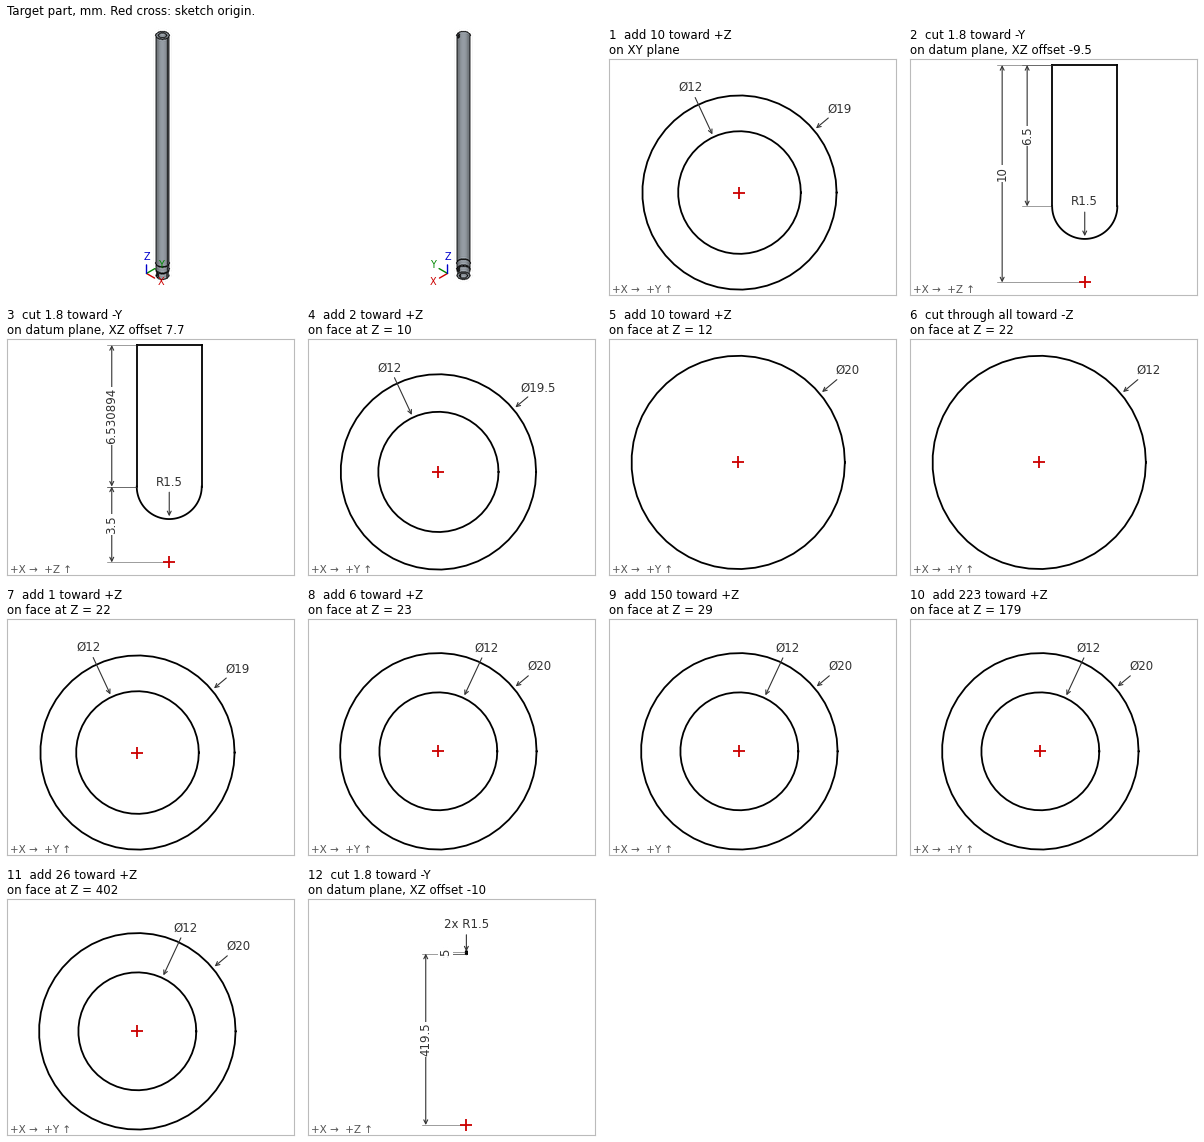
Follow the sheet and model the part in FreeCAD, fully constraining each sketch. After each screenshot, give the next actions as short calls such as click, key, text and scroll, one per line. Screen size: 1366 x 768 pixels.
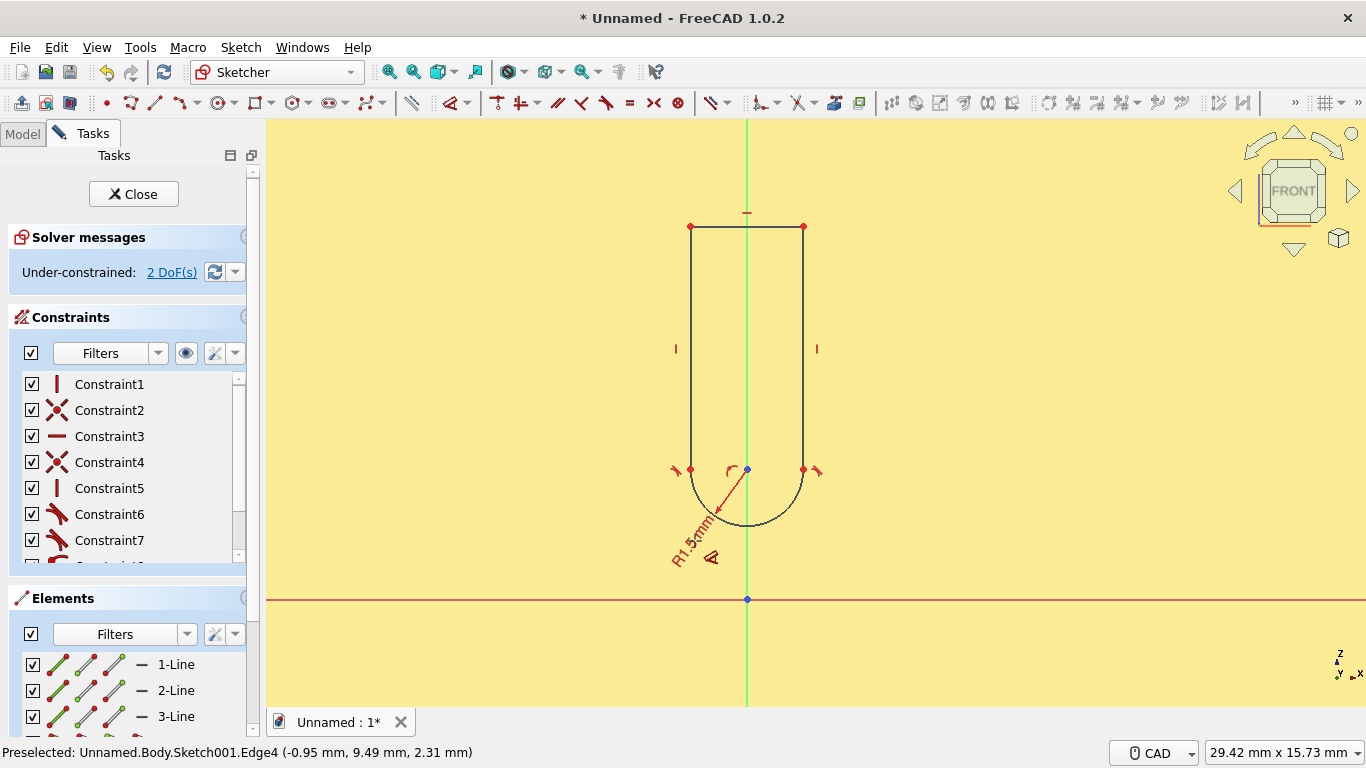
click(691, 397)
click(657, 349)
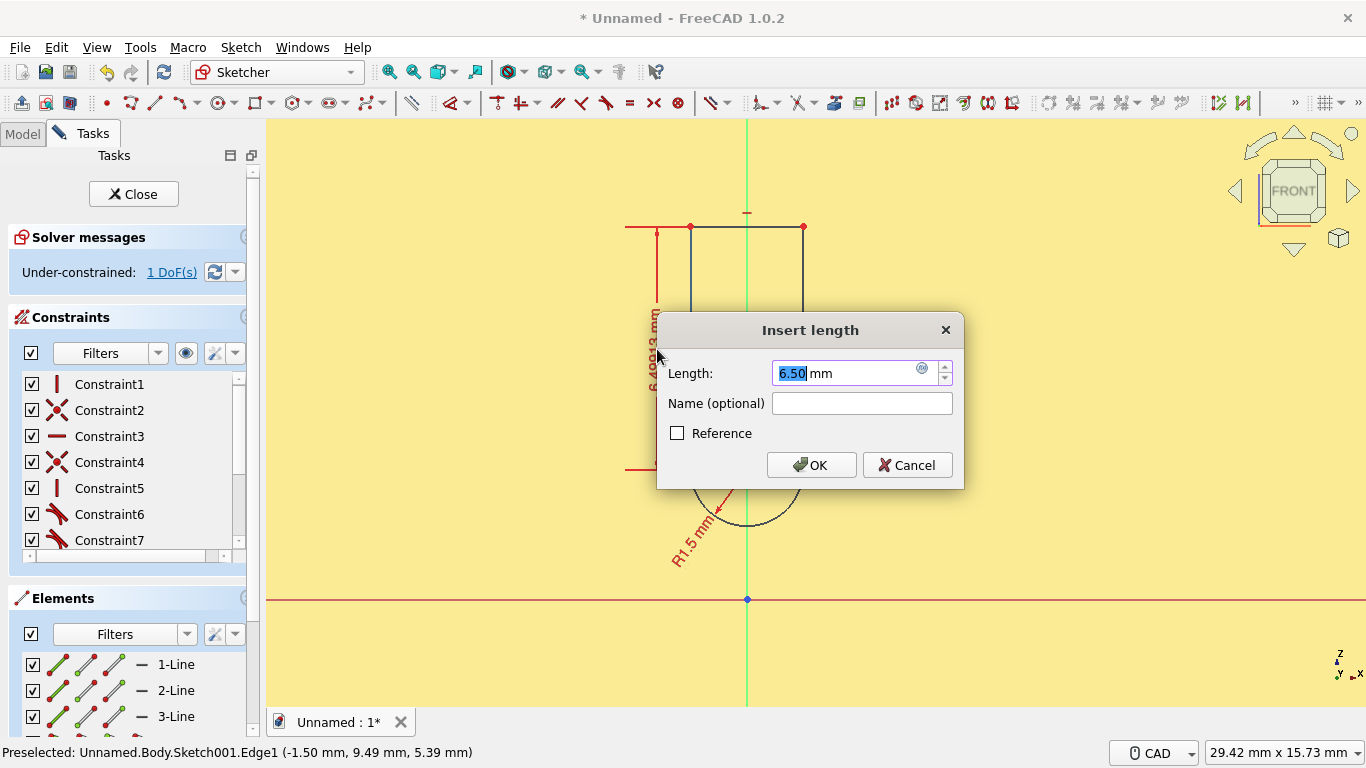
text(6.5)
key(Return)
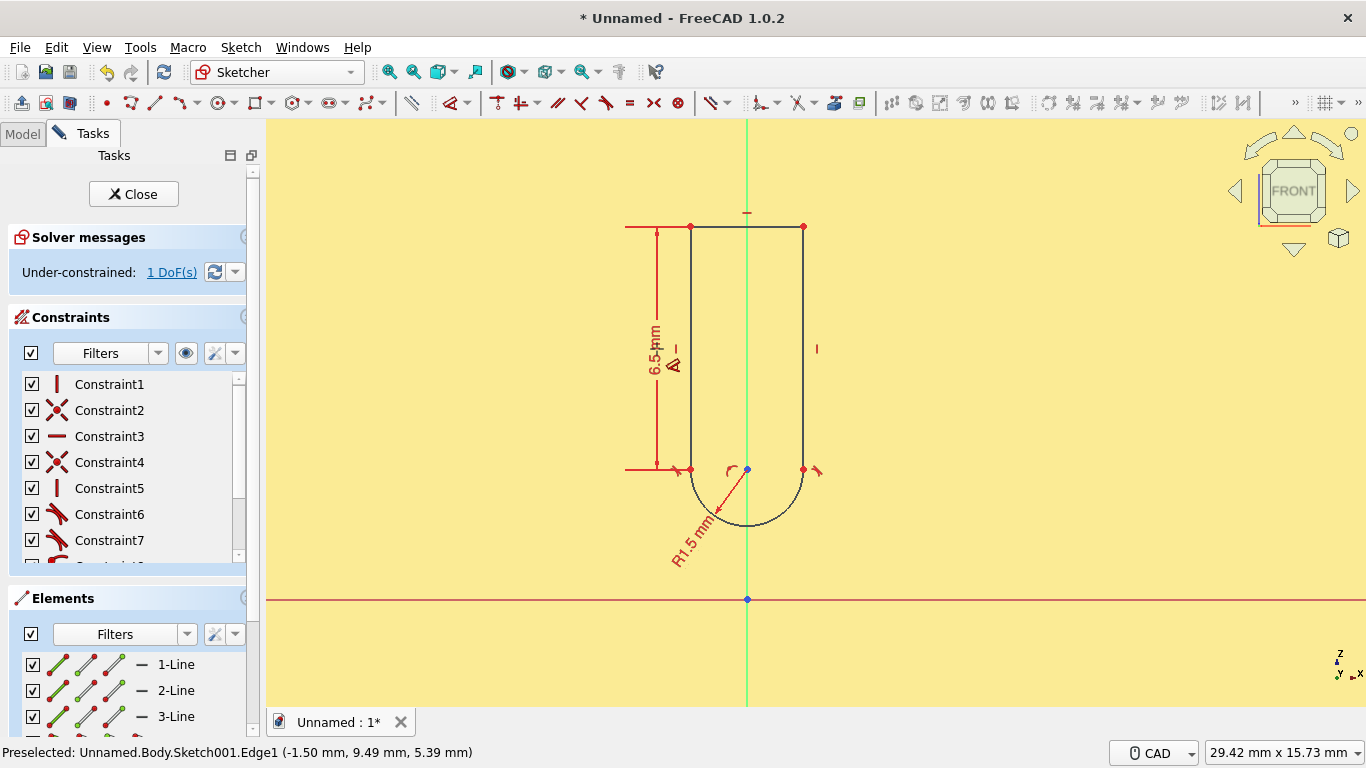
click(691, 227)
click(657, 413)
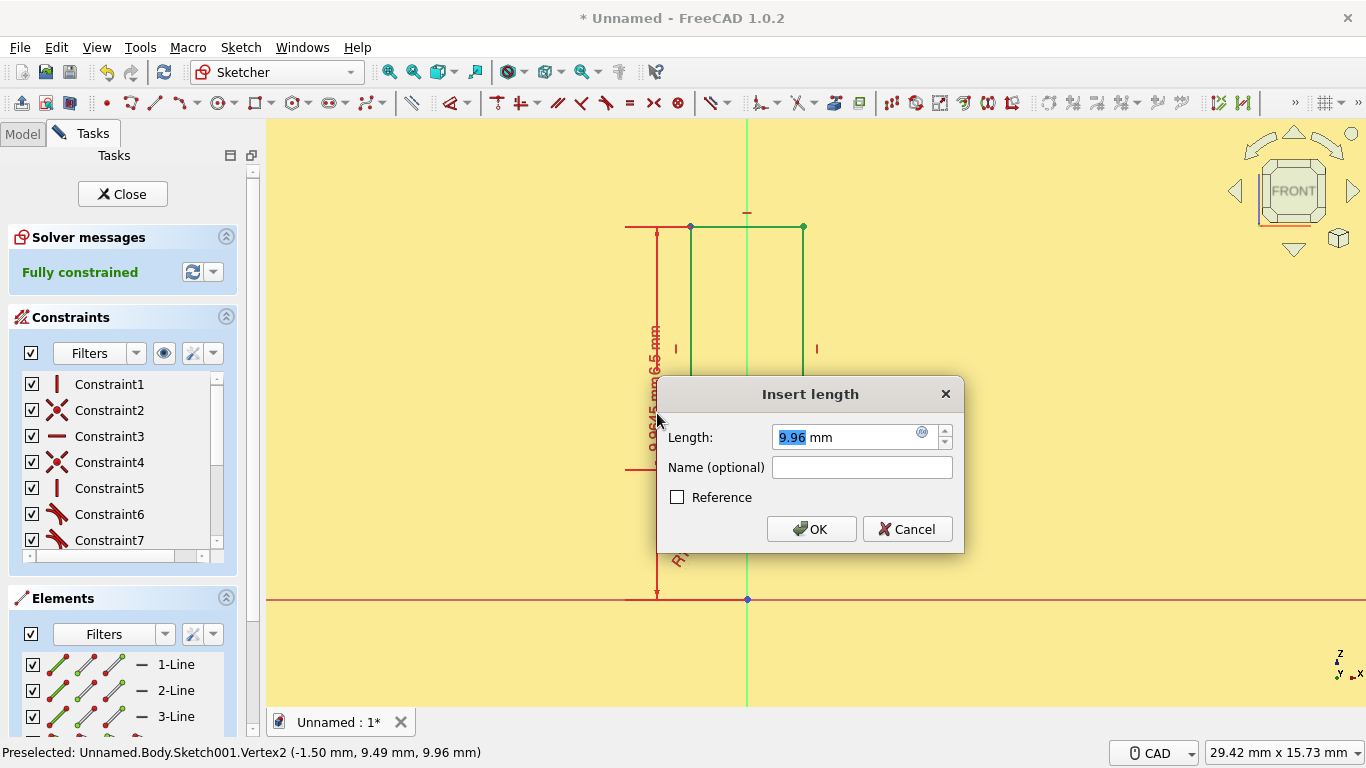
text(10)
key(Return)
key(Escape)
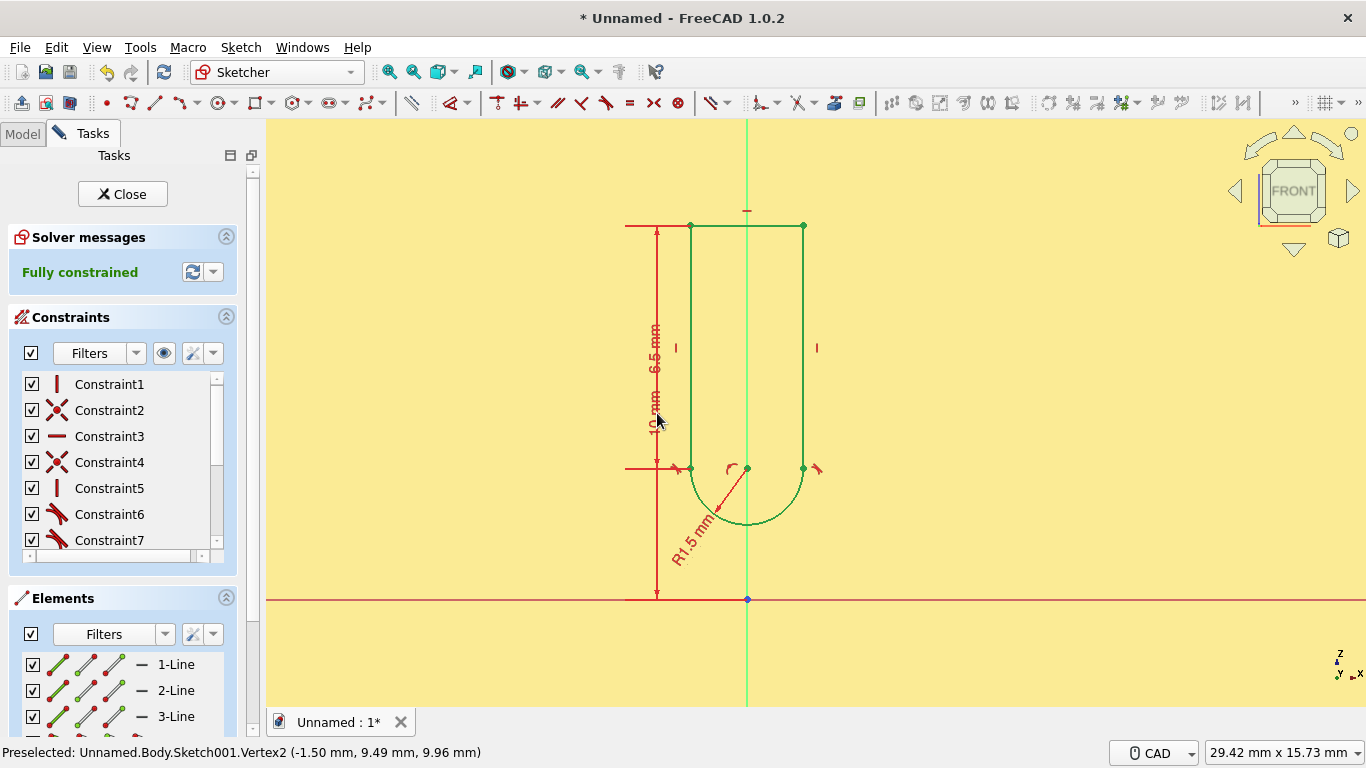
click(123, 194)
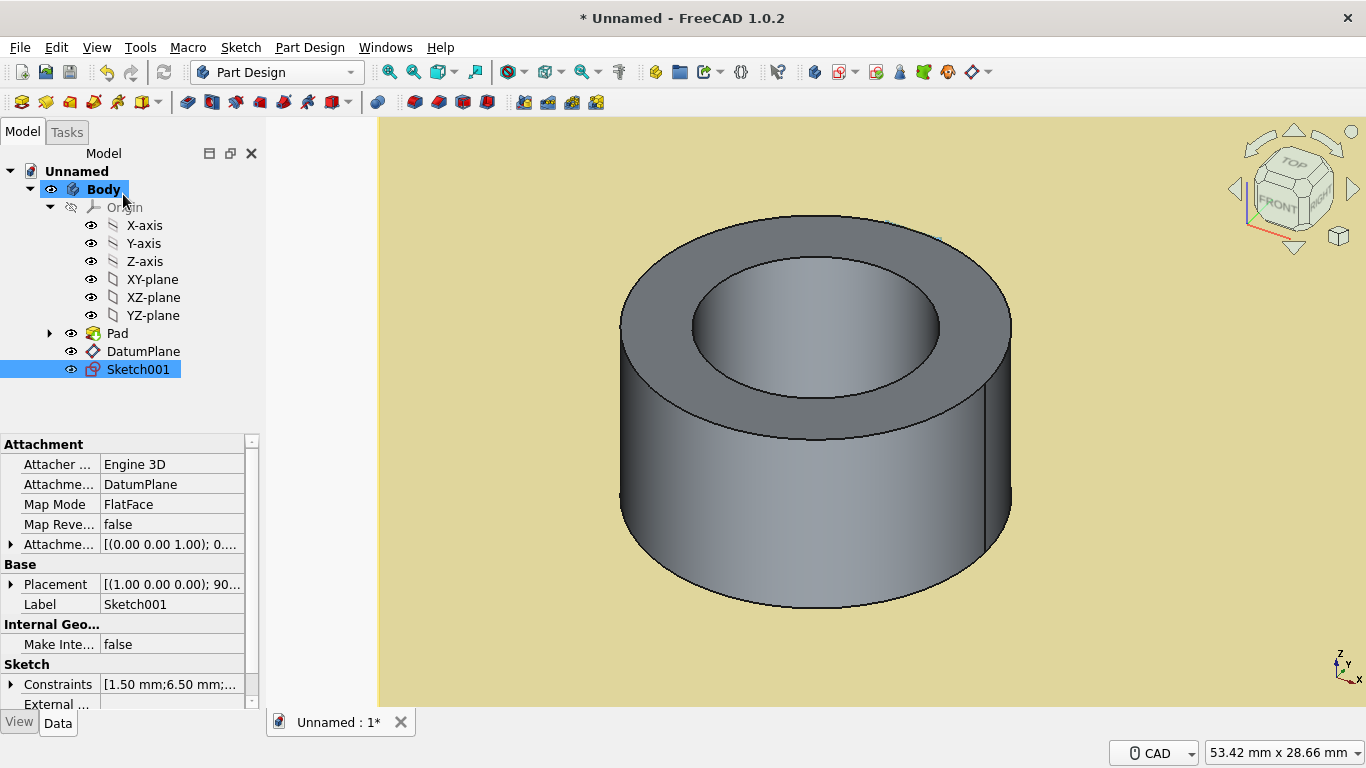
click(188, 102)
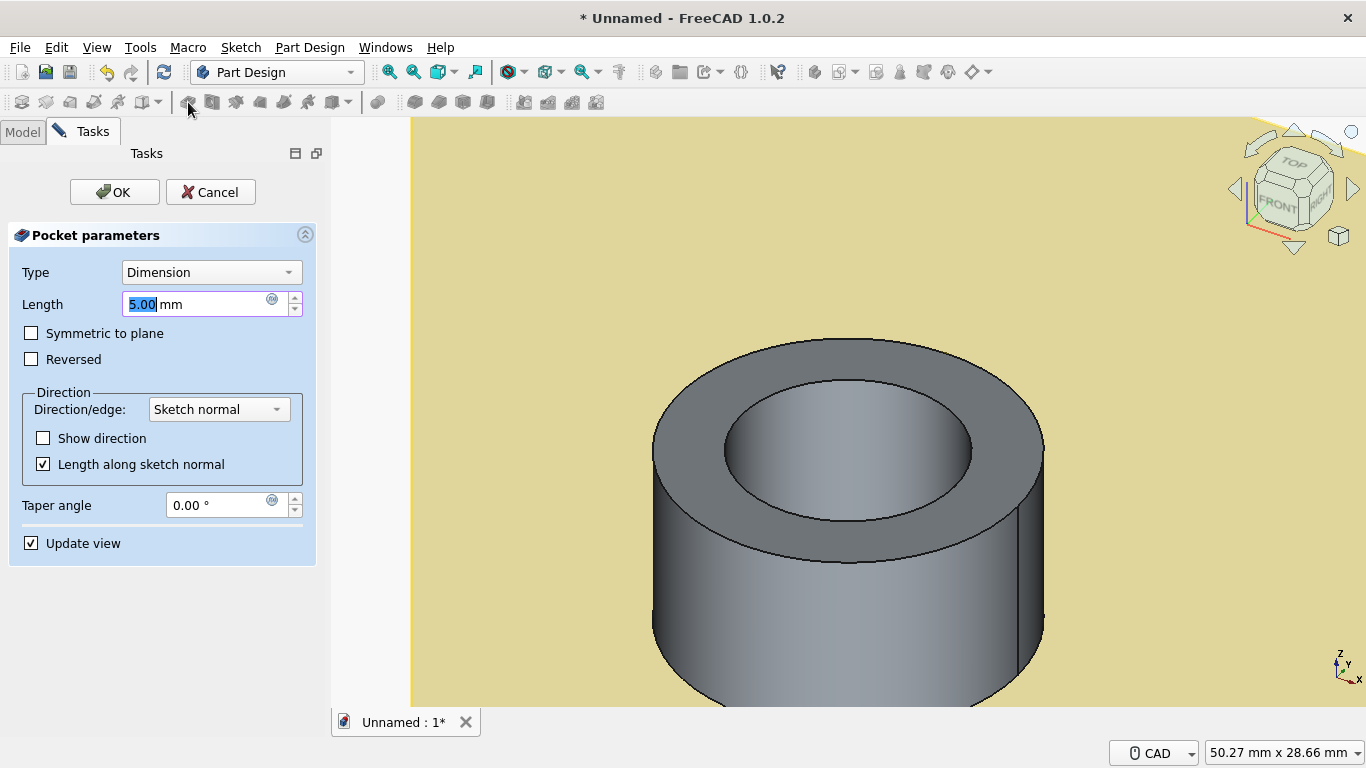
text(1.8)
key(Tab)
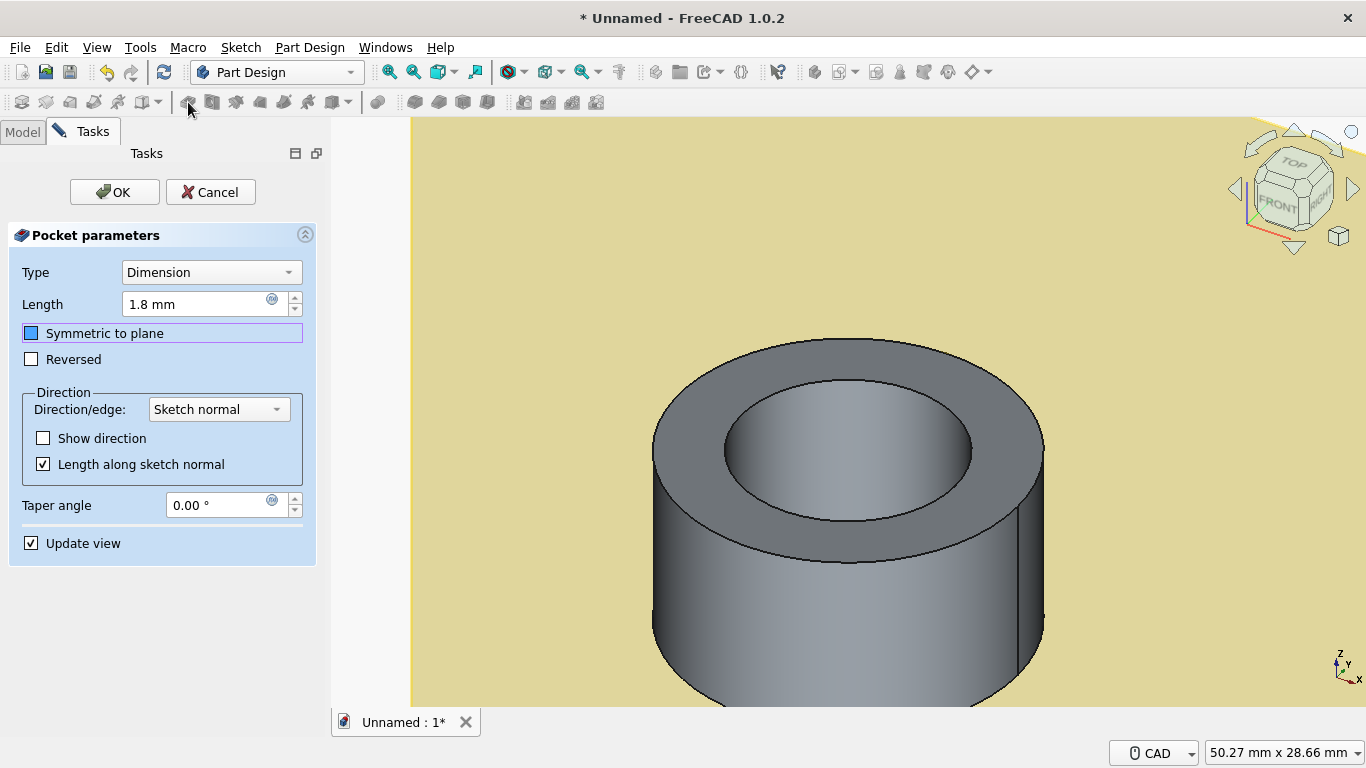
click(30, 359)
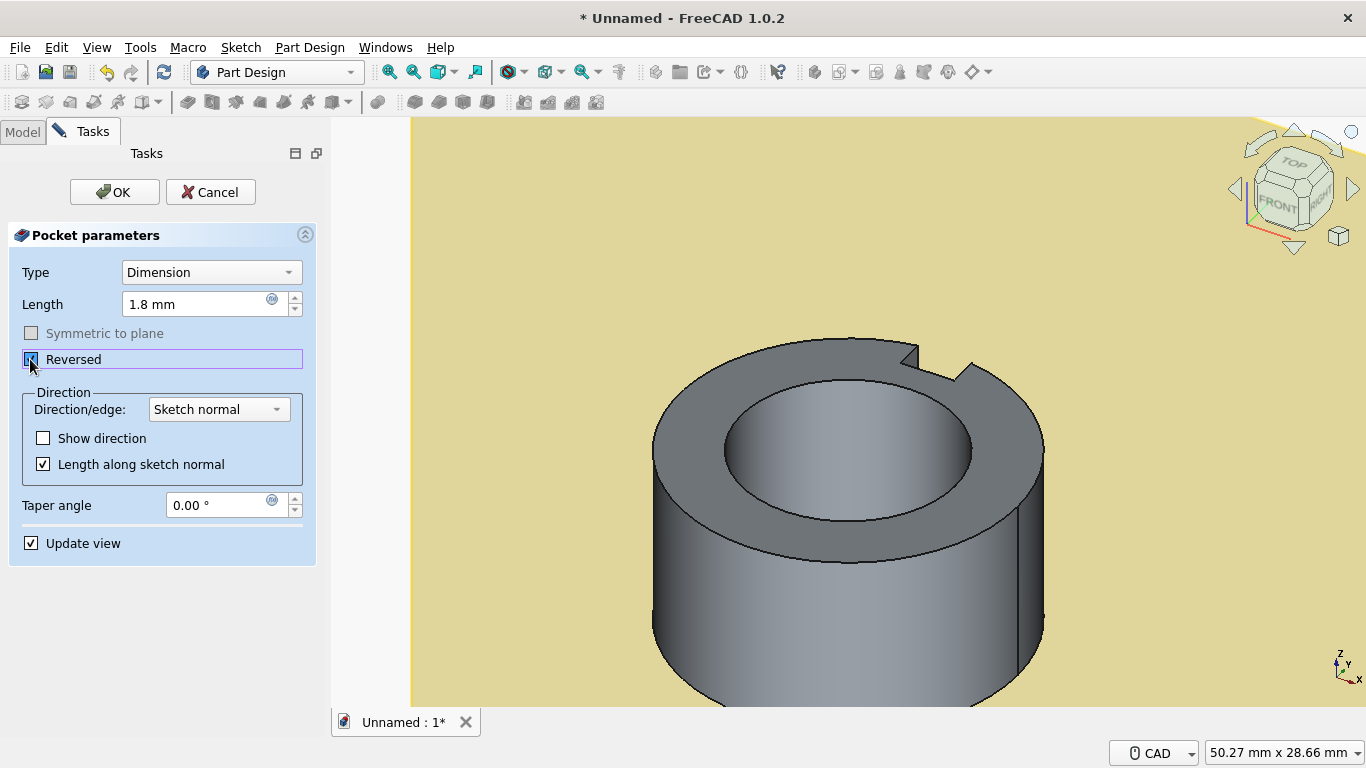
click(115, 192)